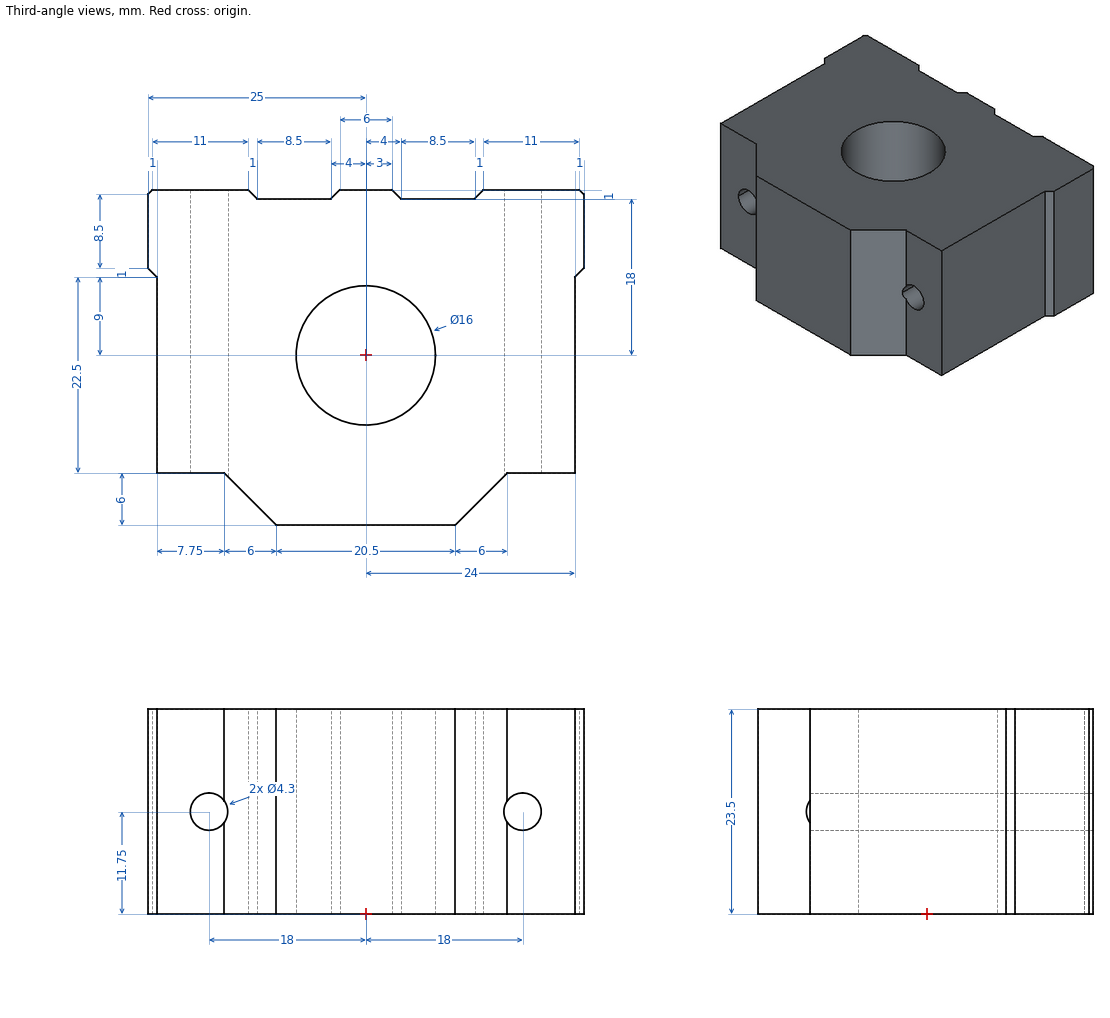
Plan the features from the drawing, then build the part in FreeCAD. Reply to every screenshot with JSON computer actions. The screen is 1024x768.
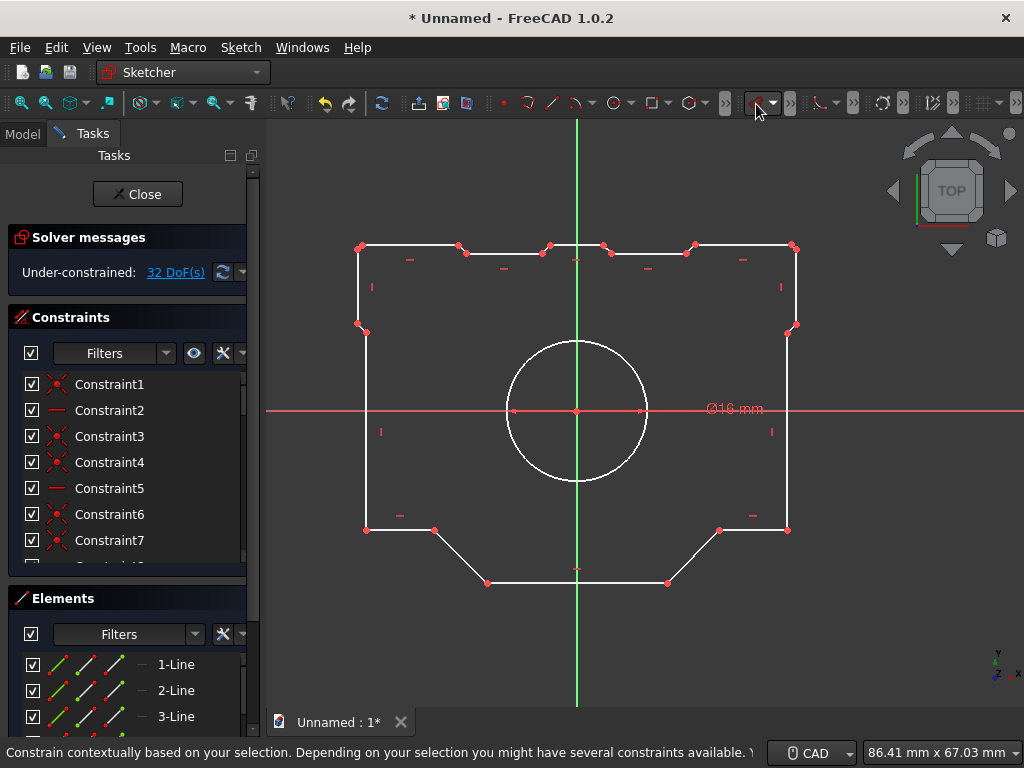
{"action": "scroll", "coordinate": [587, 245], "scroll_direction": "up", "scroll_amount": 2}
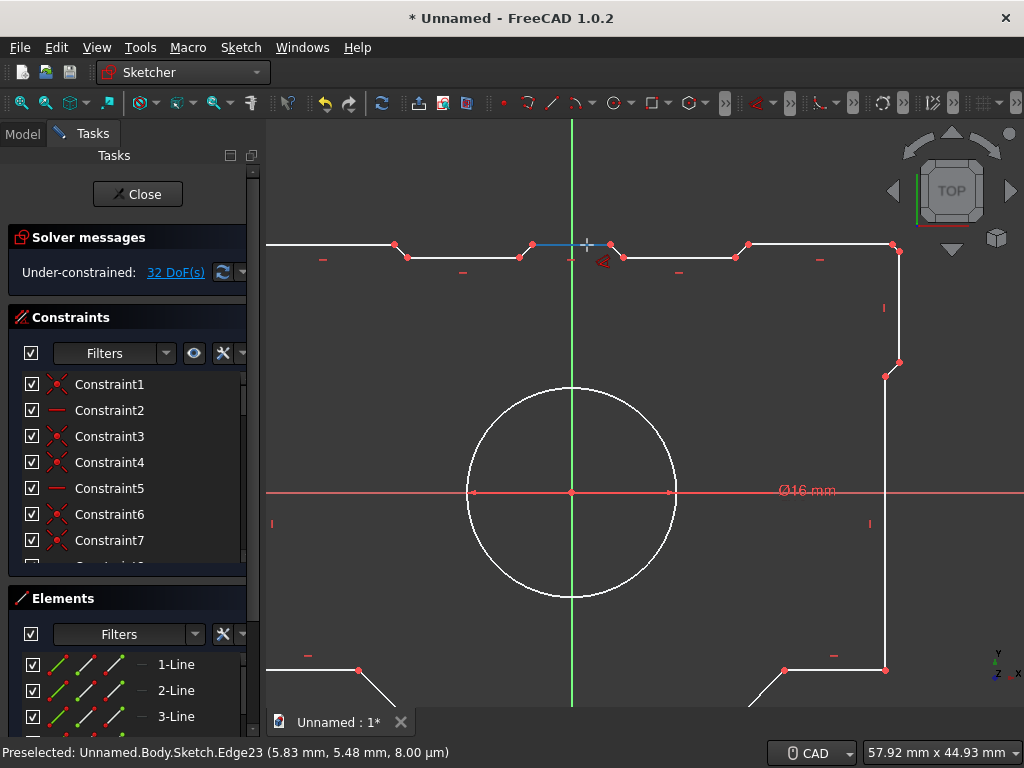
{"action": "left_click", "coordinate": [587, 245]}
{"action": "left_click", "coordinate": [554, 211]}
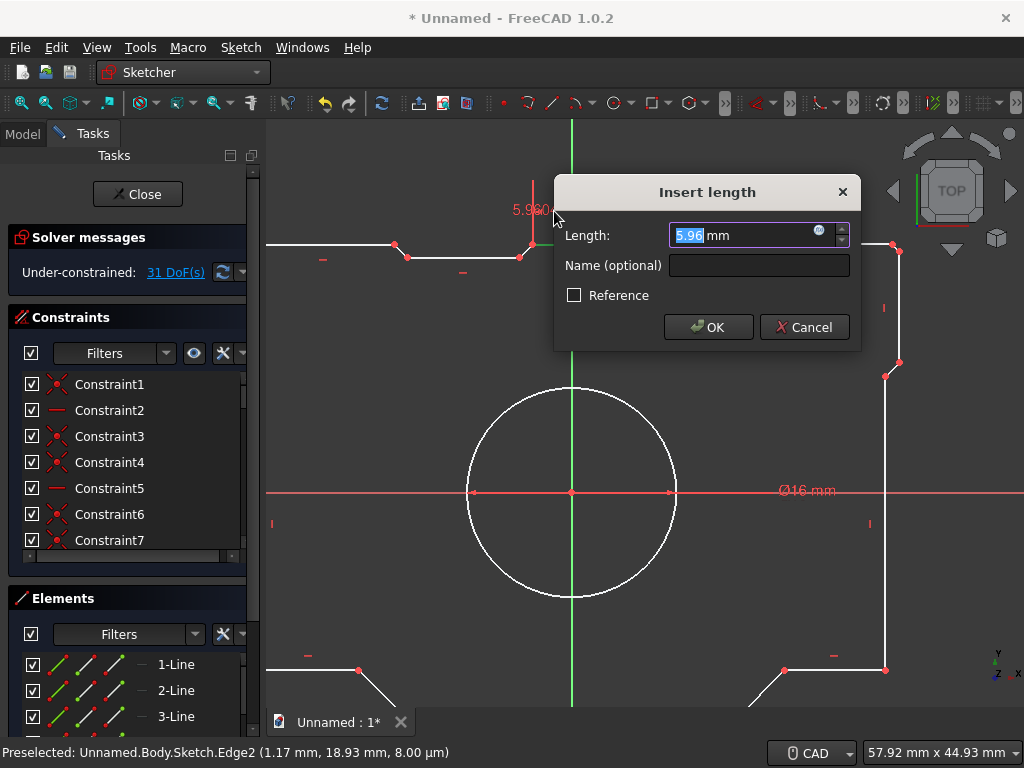
{"action": "type", "text": "6"}
{"action": "key", "text": "Return"}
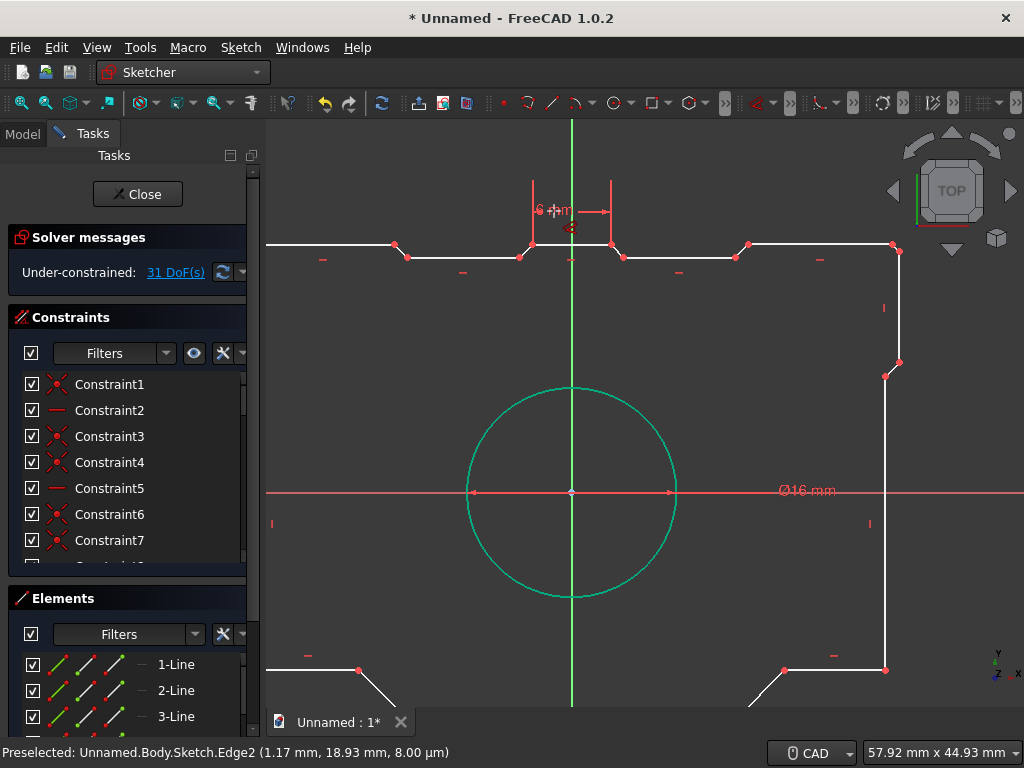
{"action": "left_click", "coordinate": [352, 245]}
{"action": "left_click", "coordinate": [344, 211]}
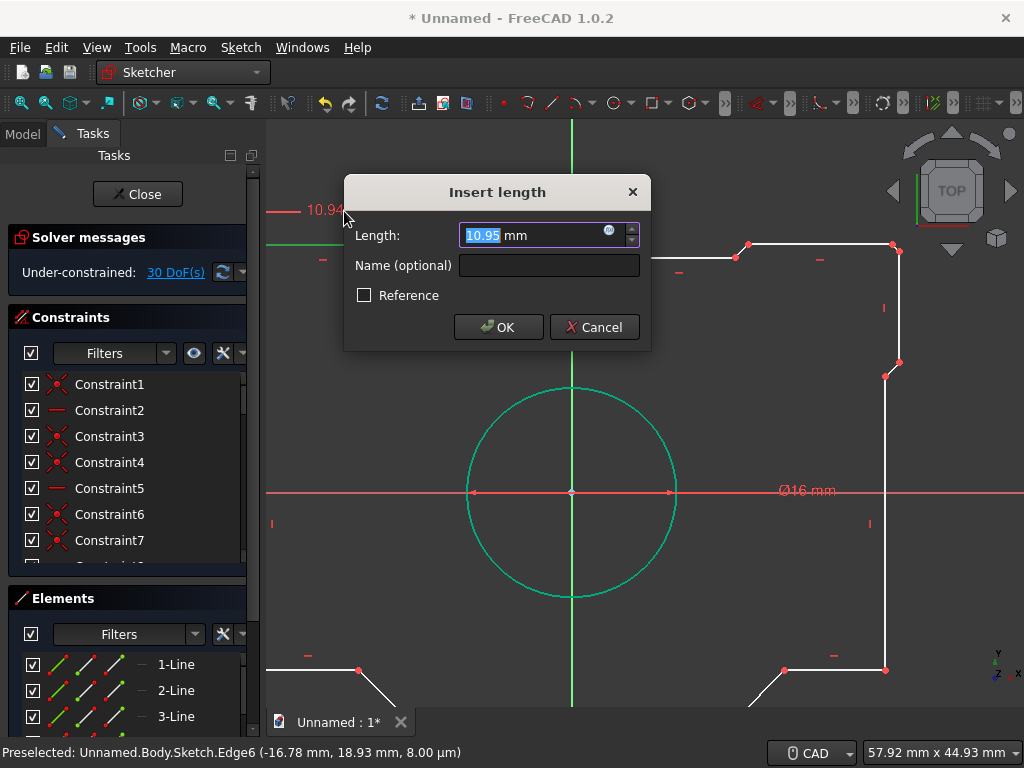
{"action": "type", "text": "11"}
{"action": "key", "text": "Return"}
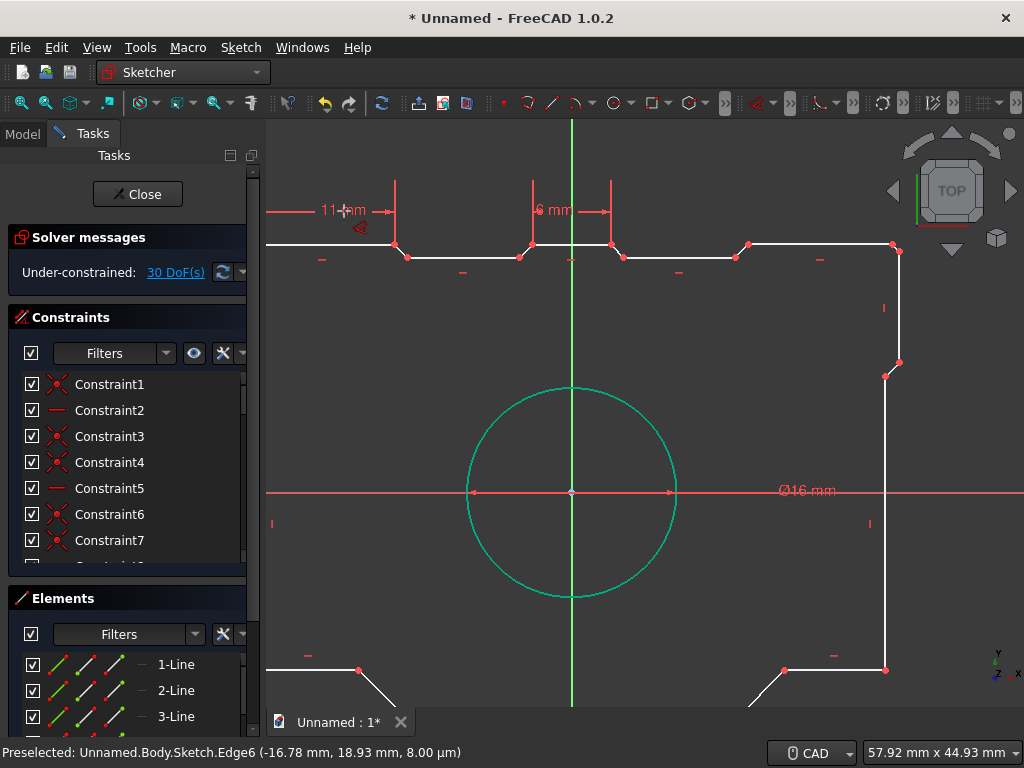
{"action": "left_click", "coordinate": [849, 244]}
{"action": "left_click", "coordinate": [804, 210]}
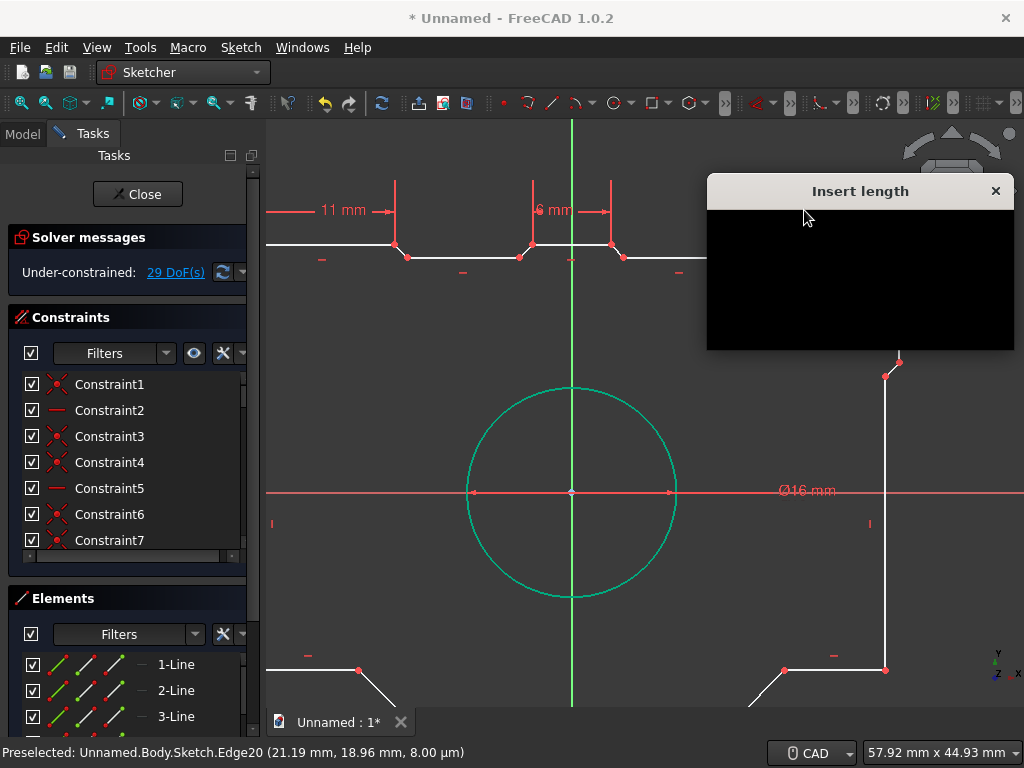
{"action": "type", "text": "11"}
{"action": "key", "text": "Return"}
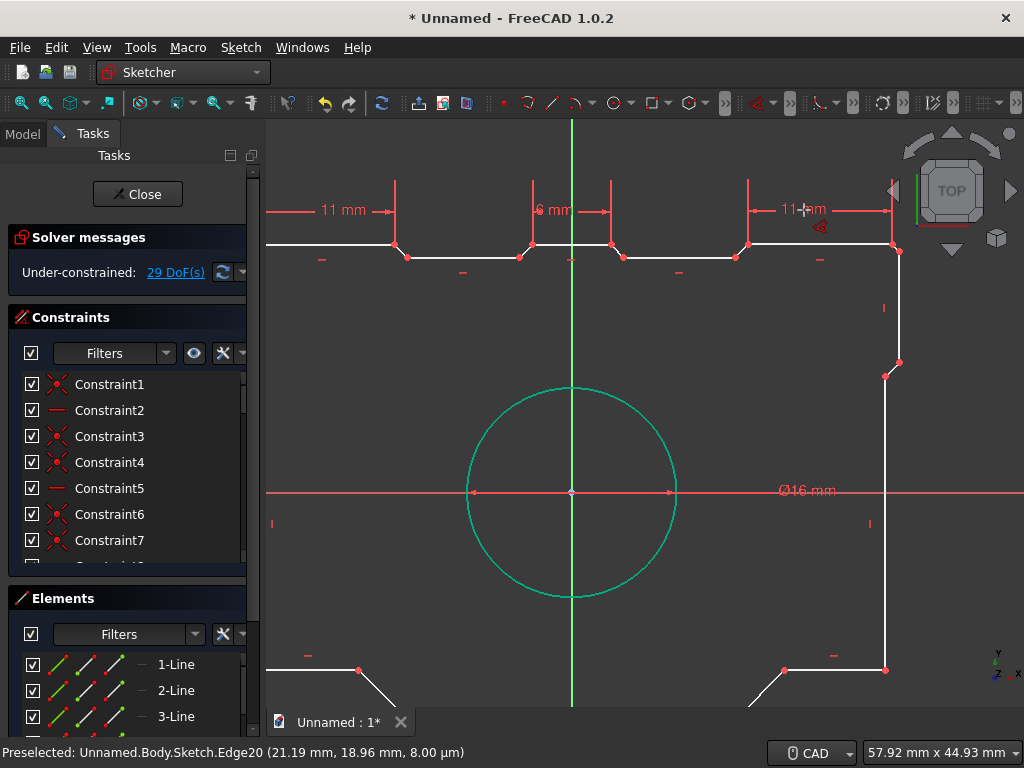
{"action": "left_click", "coordinate": [623, 258]}
{"action": "left_click", "coordinate": [598, 527]}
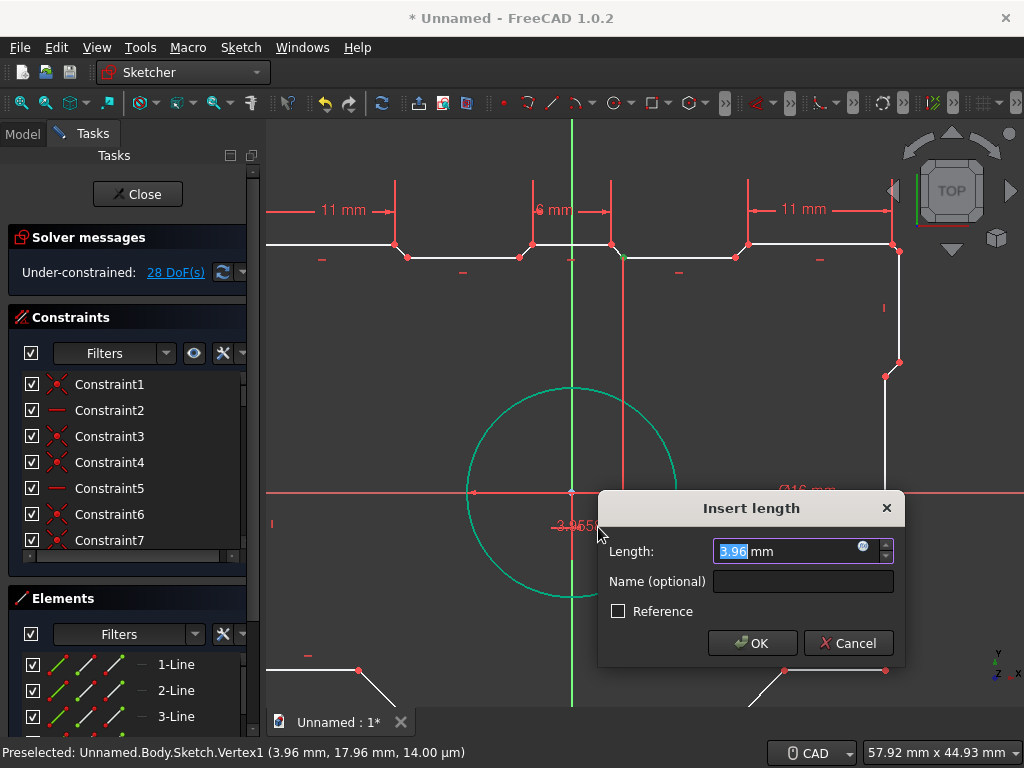
{"action": "type", "text": "4"}
{"action": "key", "text": "Return"}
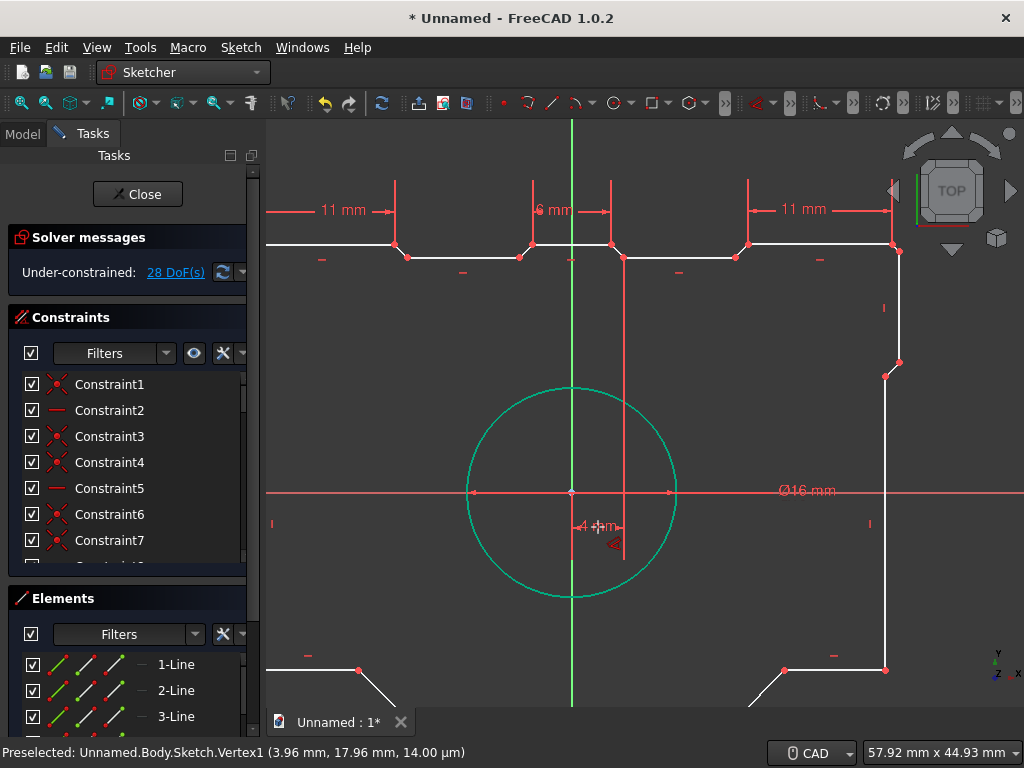
{"action": "left_click", "coordinate": [611, 245]}
{"action": "left_click", "coordinate": [591, 187]}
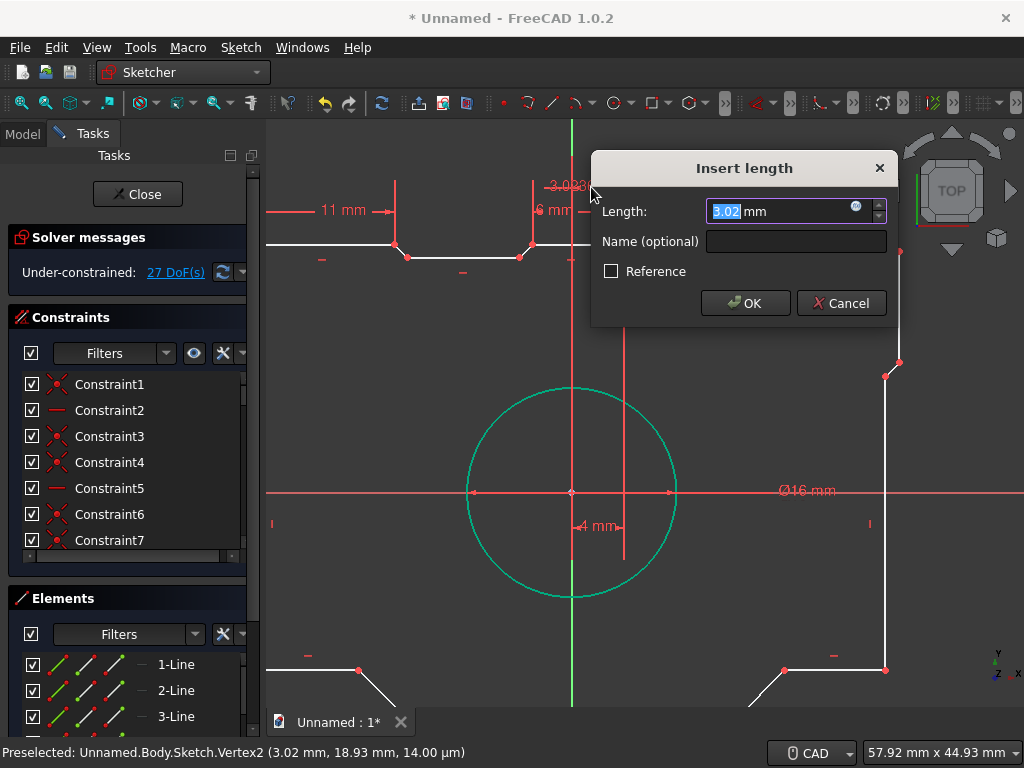
{"action": "type", "text": "3"}
{"action": "key", "text": "Return"}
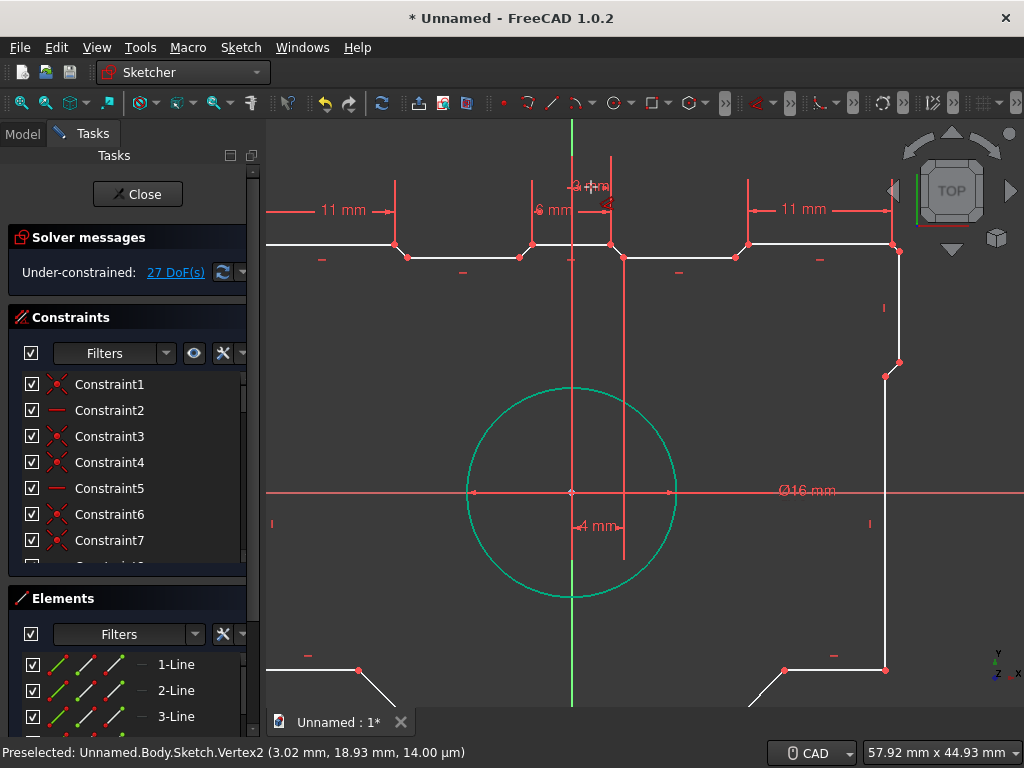
{"action": "left_click", "coordinate": [520, 258]}
{"action": "left_click", "coordinate": [527, 527]}